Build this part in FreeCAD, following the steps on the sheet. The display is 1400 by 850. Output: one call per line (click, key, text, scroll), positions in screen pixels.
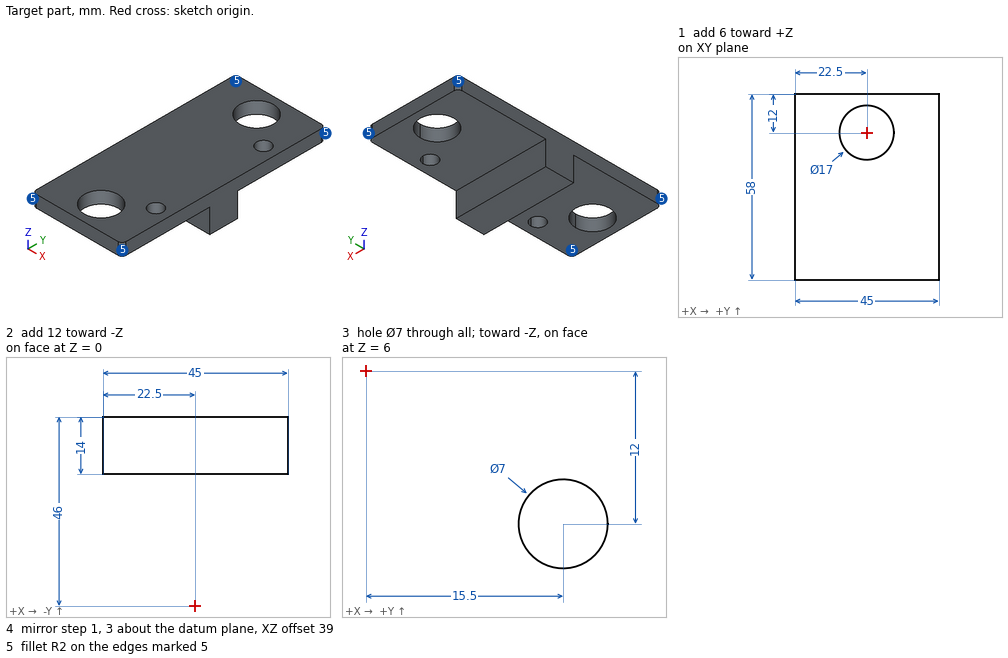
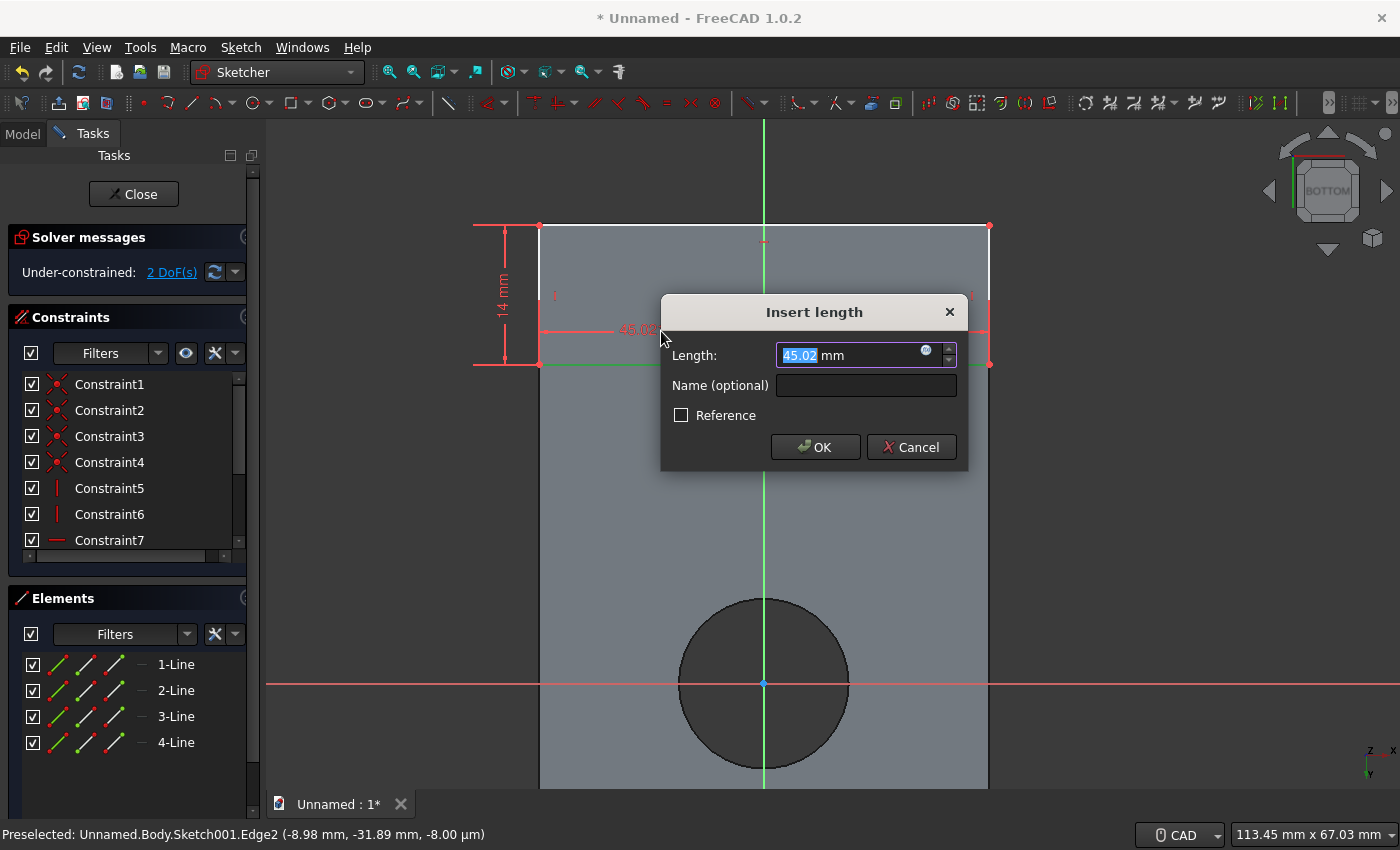
text(45)
key(Return)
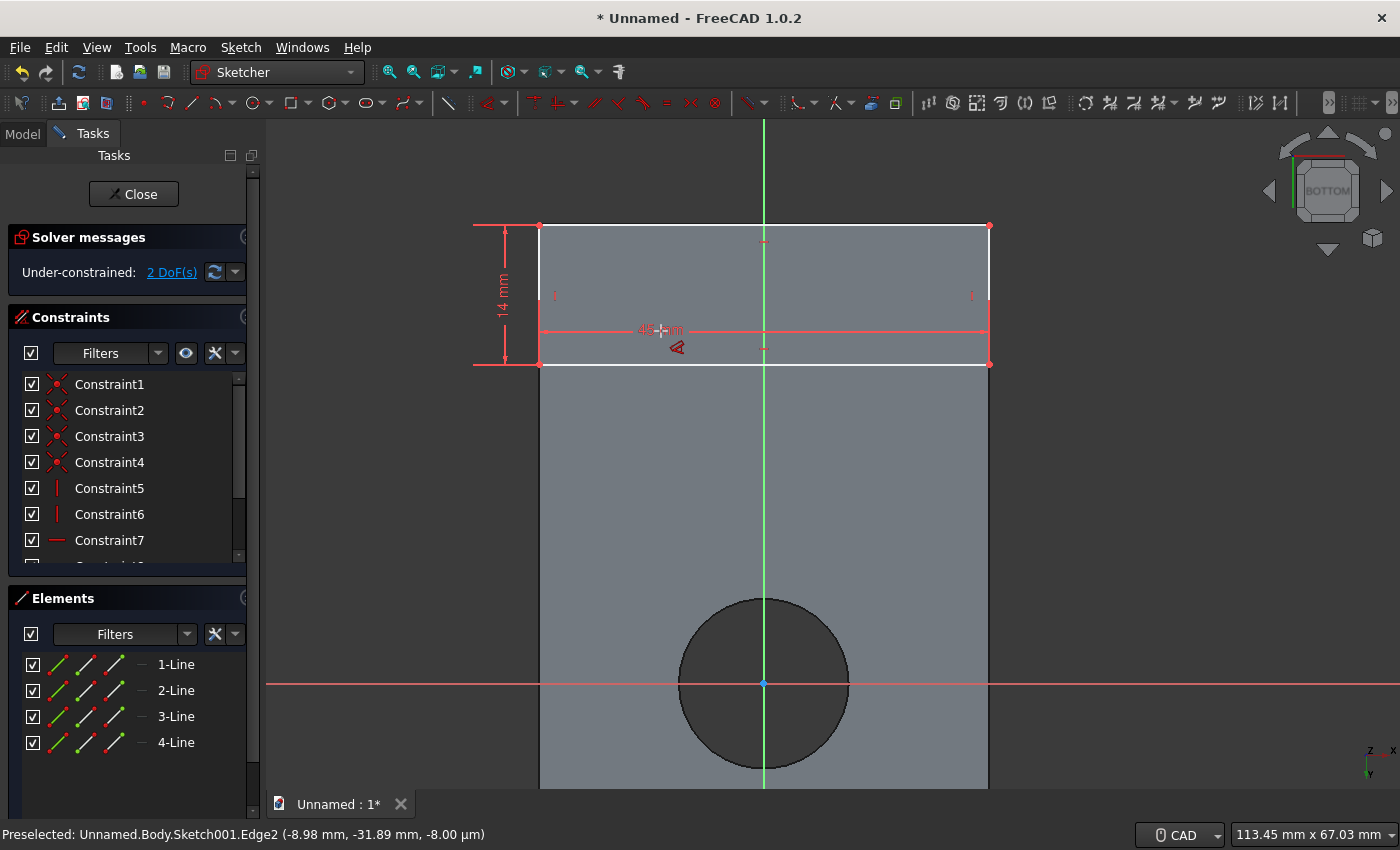
click(539, 225)
click(505, 454)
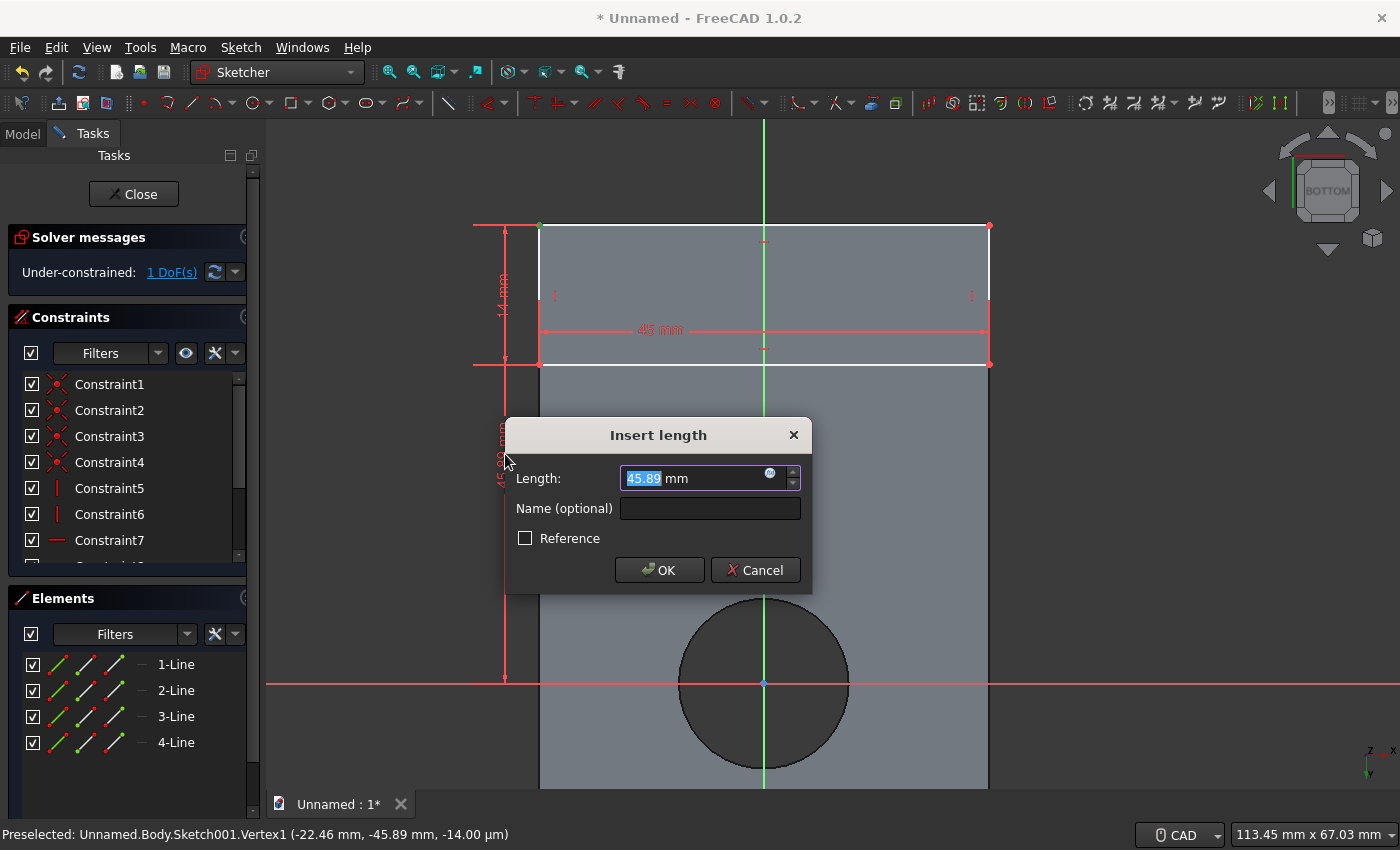
text(46)
key(Return)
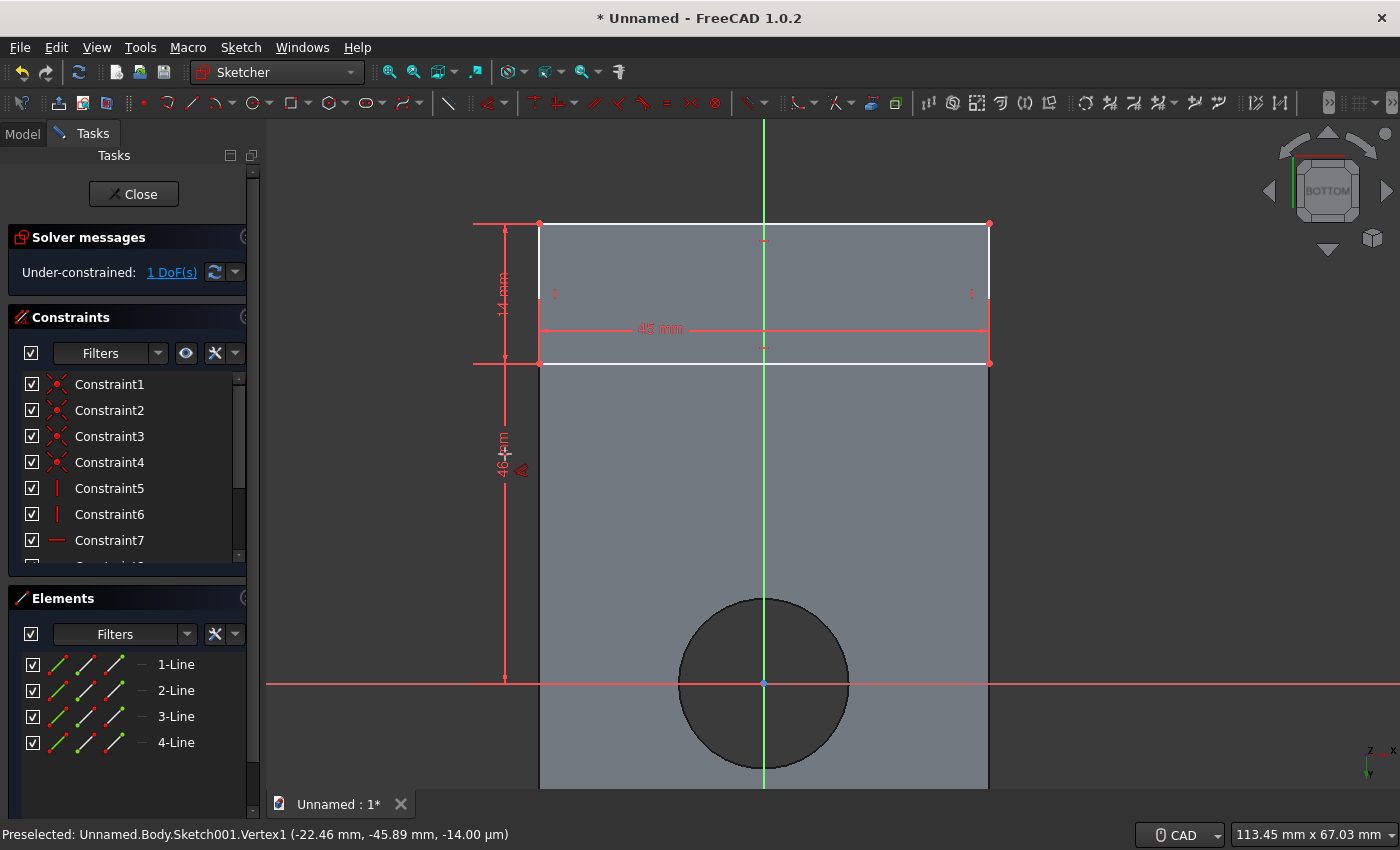
click(539, 224)
click(651, 718)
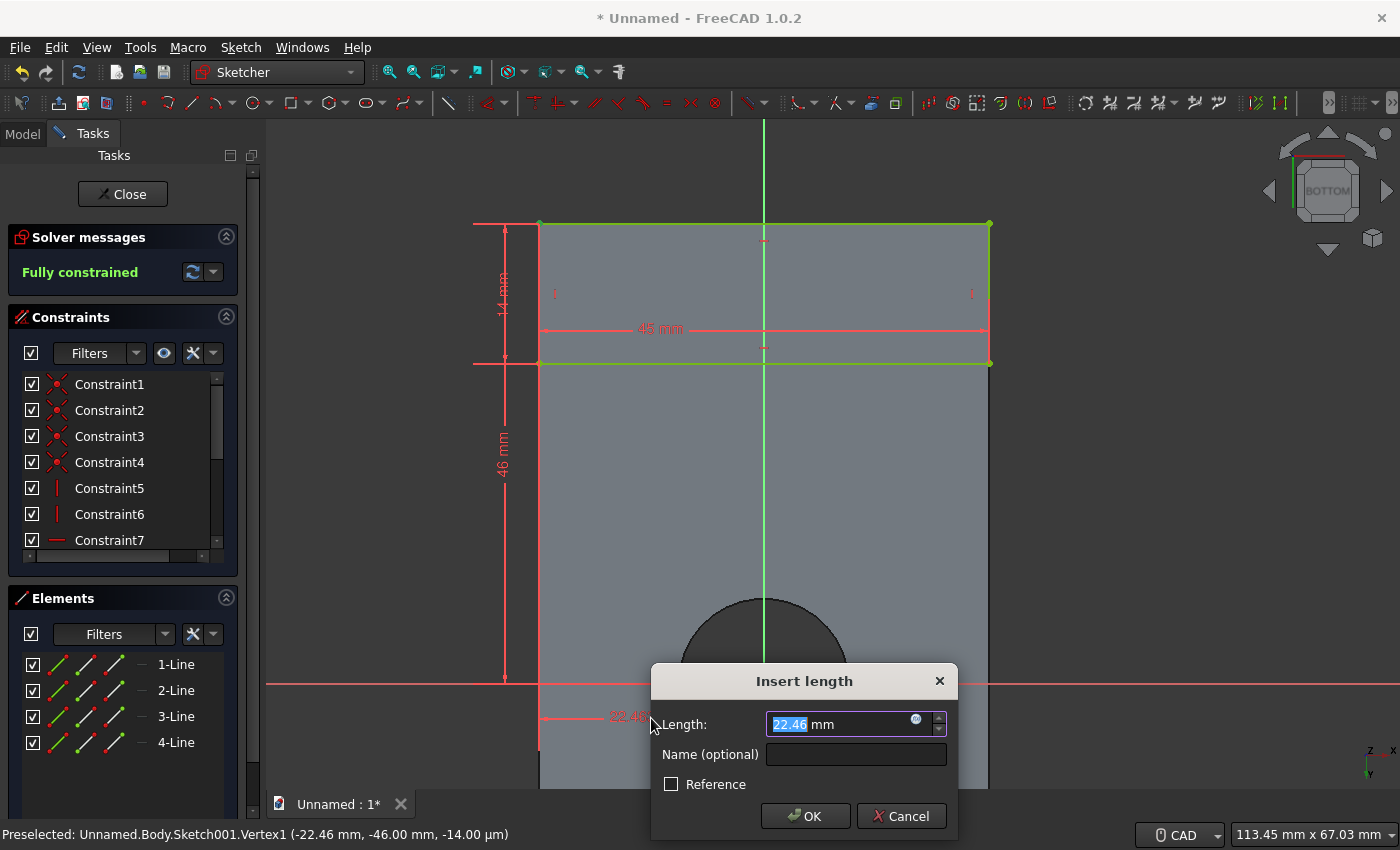
text(22.5)
key(Return)
key(Escape)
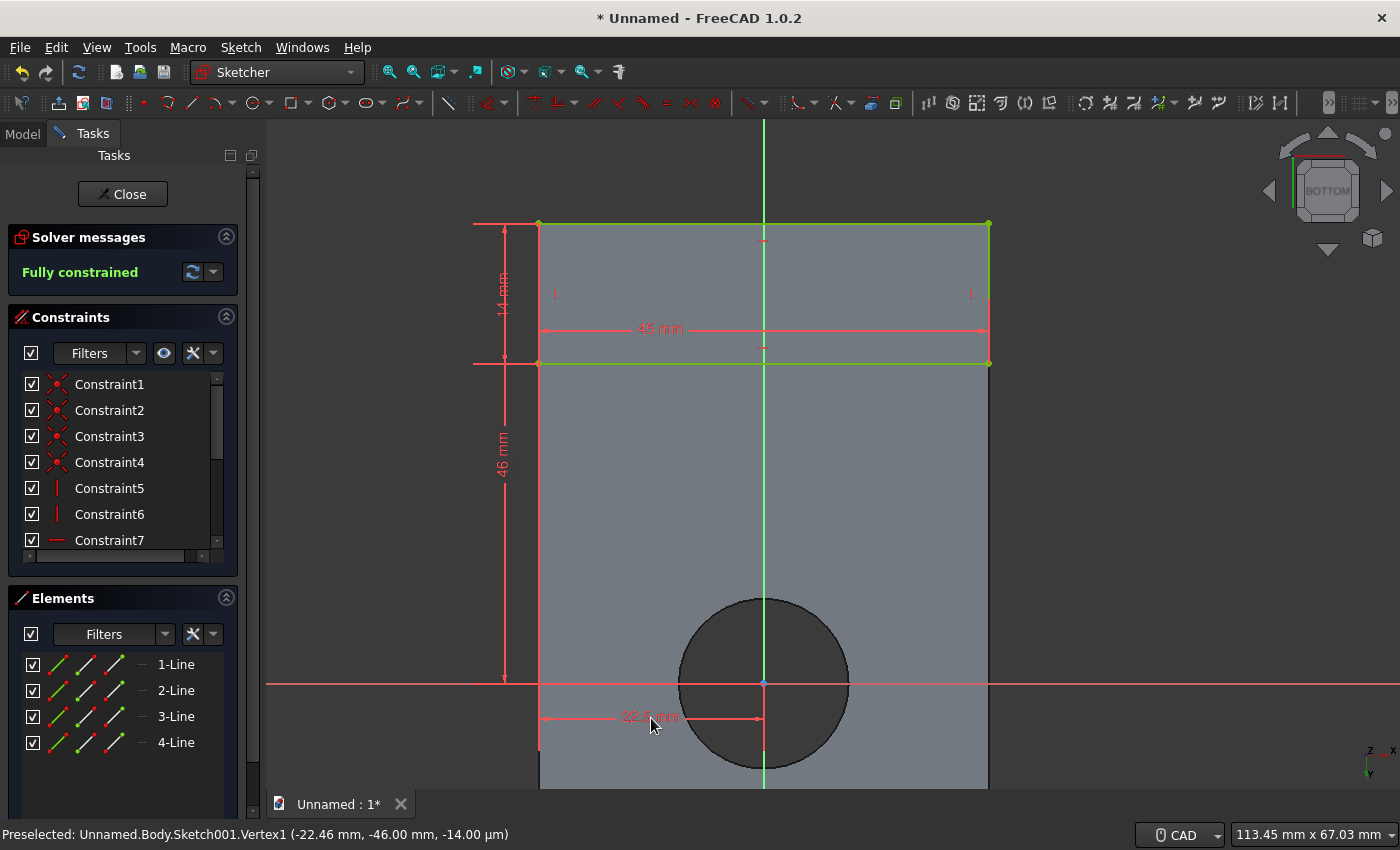
click(123, 194)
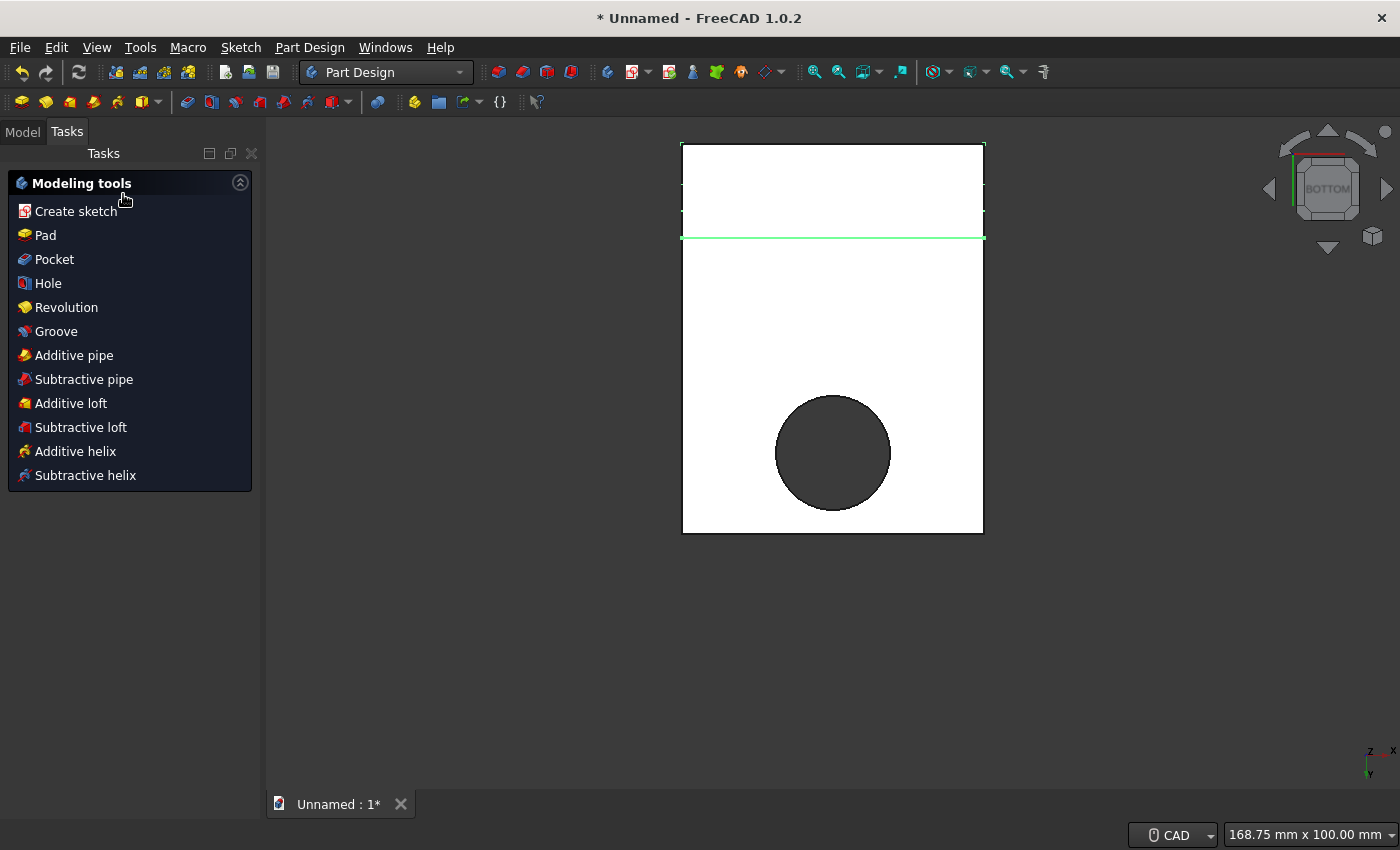
click(22, 102)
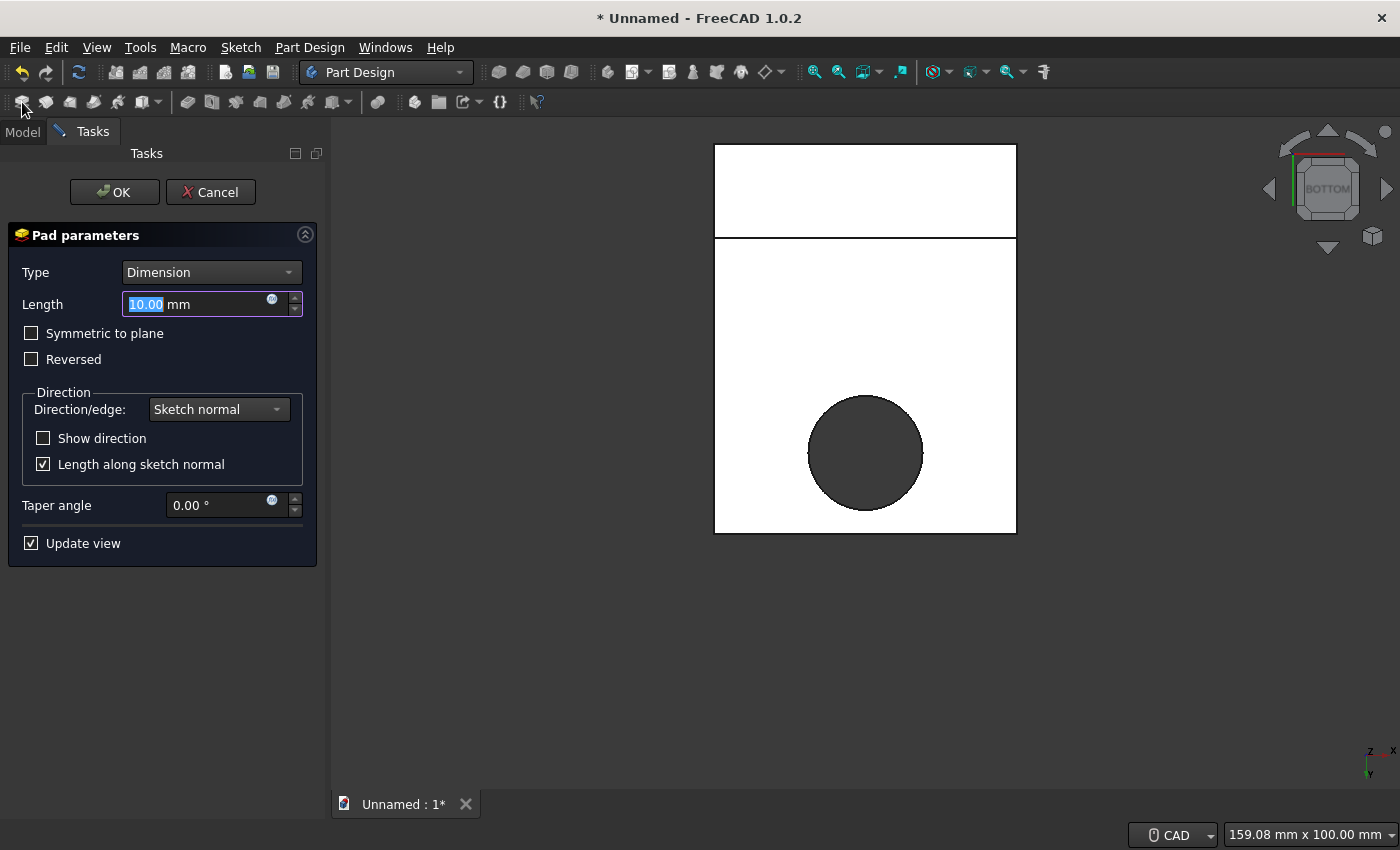
text(12)
key(Tab)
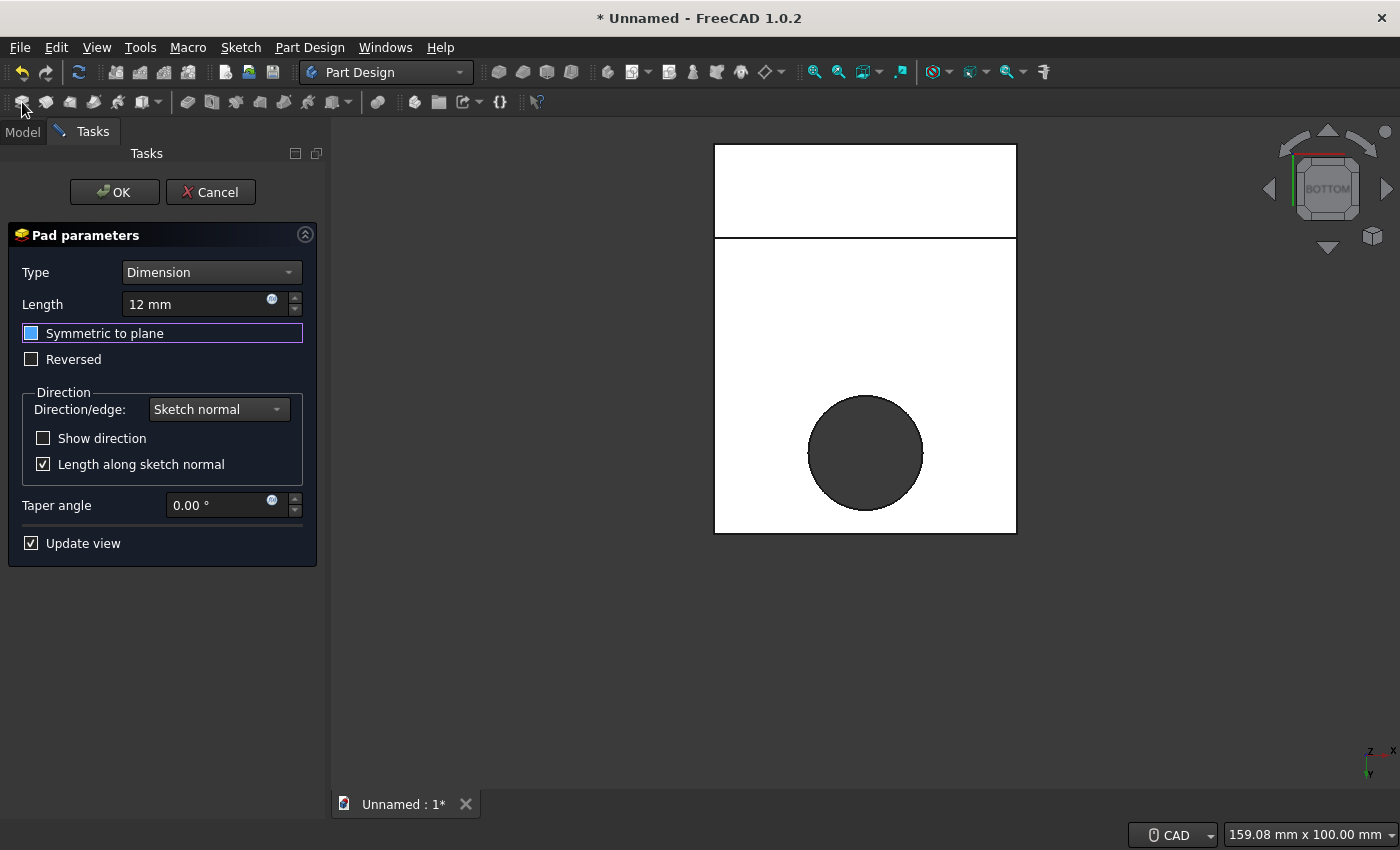
click(115, 192)